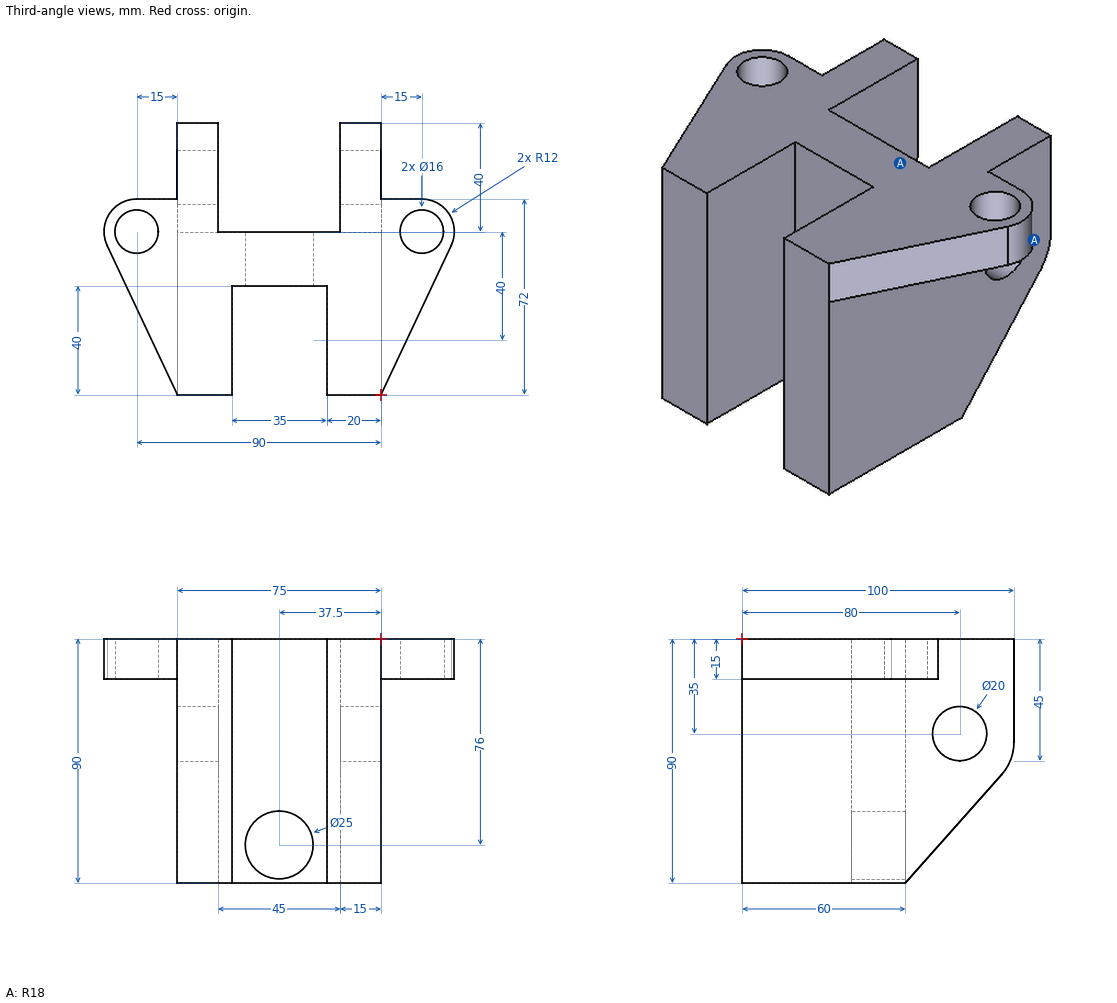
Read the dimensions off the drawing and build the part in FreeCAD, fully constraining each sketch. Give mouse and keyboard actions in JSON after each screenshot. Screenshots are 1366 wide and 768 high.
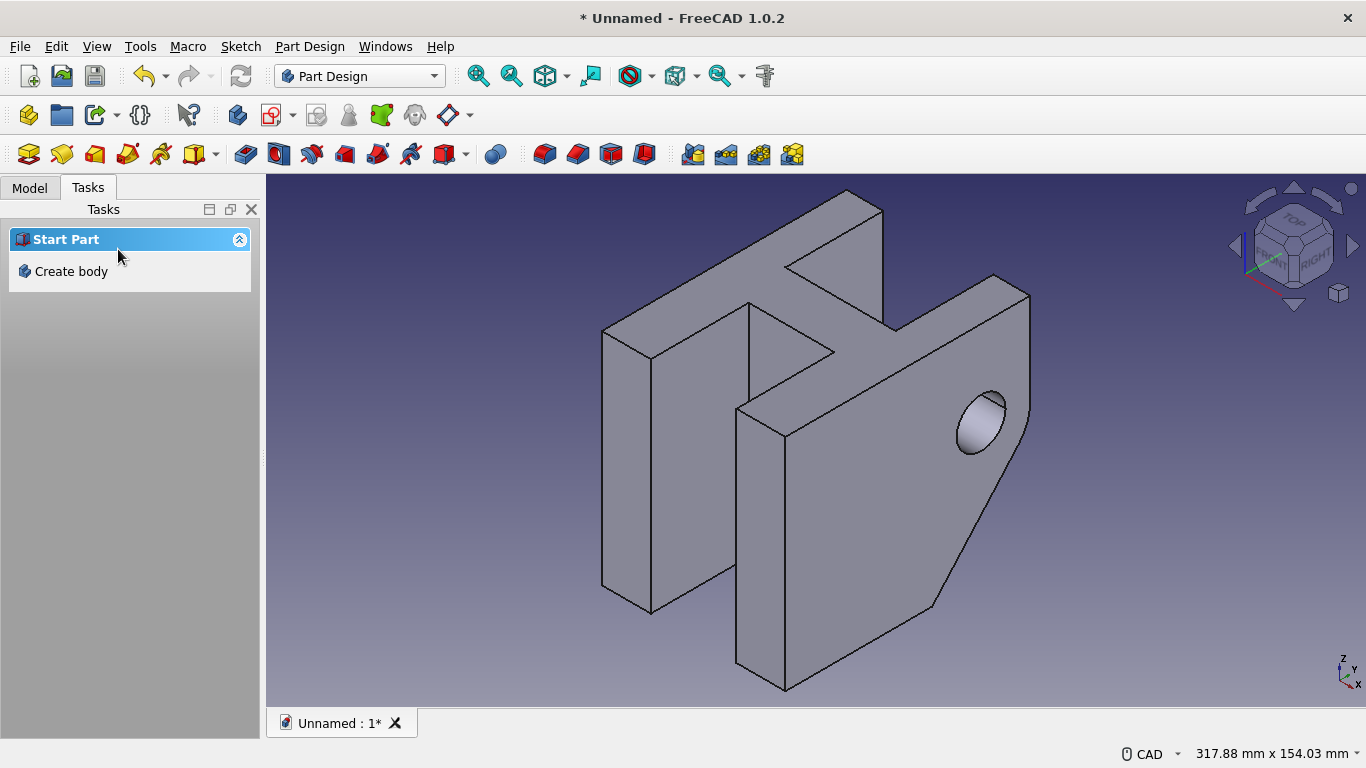
{"action": "key", "text": "4"}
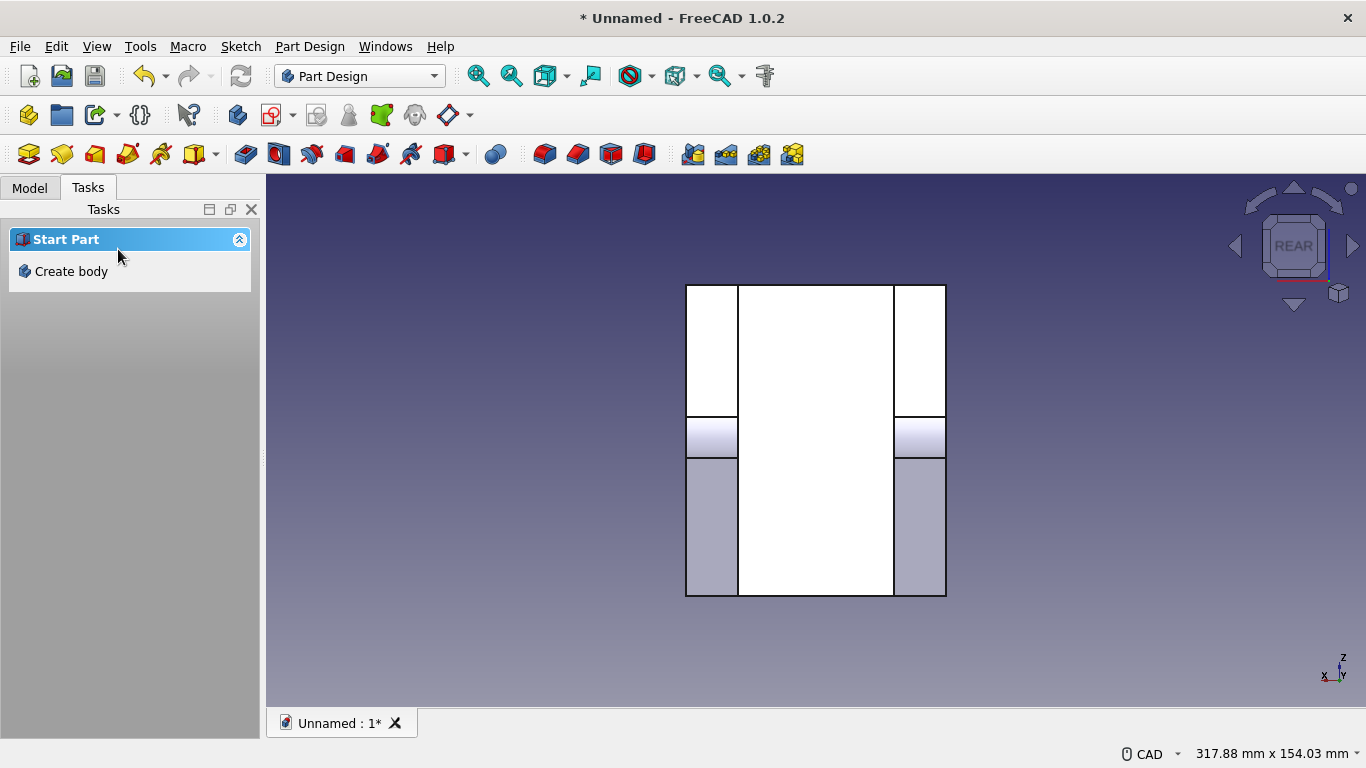
{"action": "left_click", "coordinate": [816, 484]}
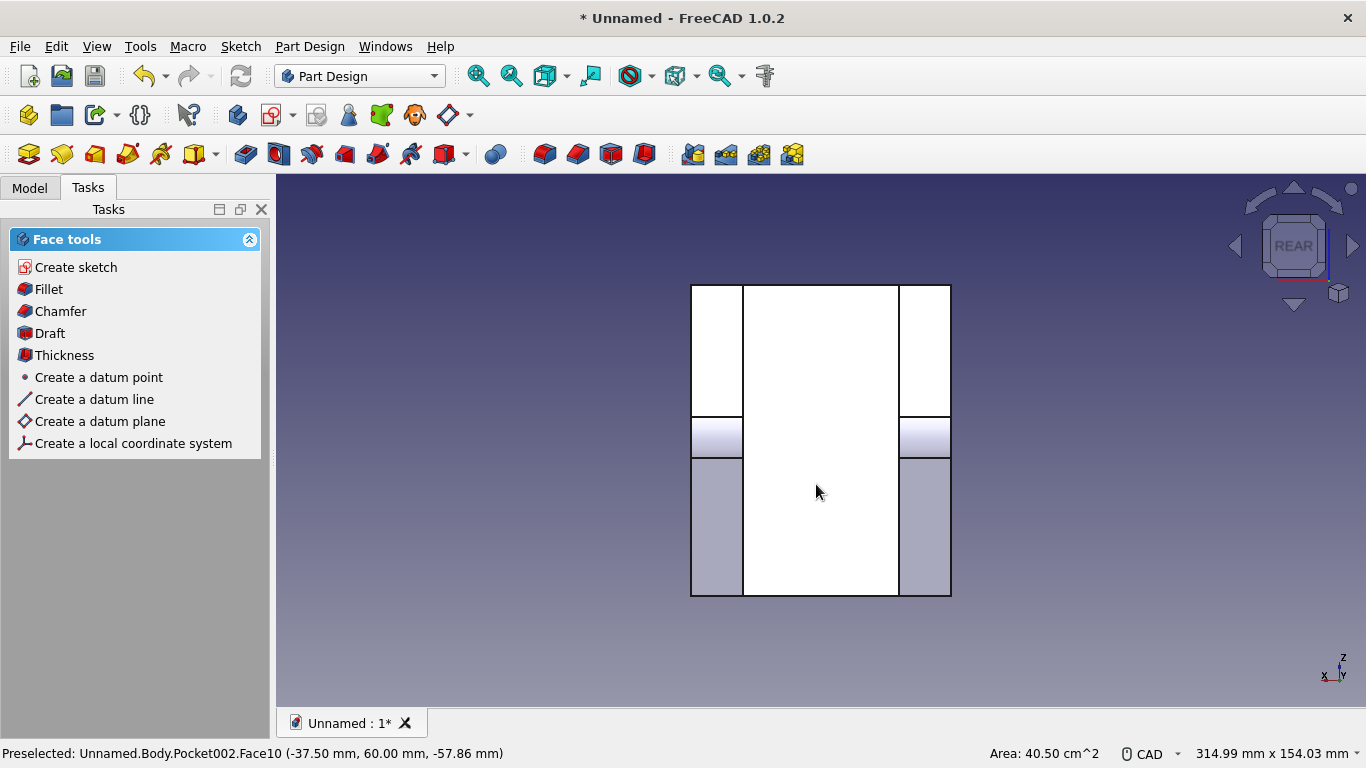
{"action": "left_click", "coordinate": [270, 116]}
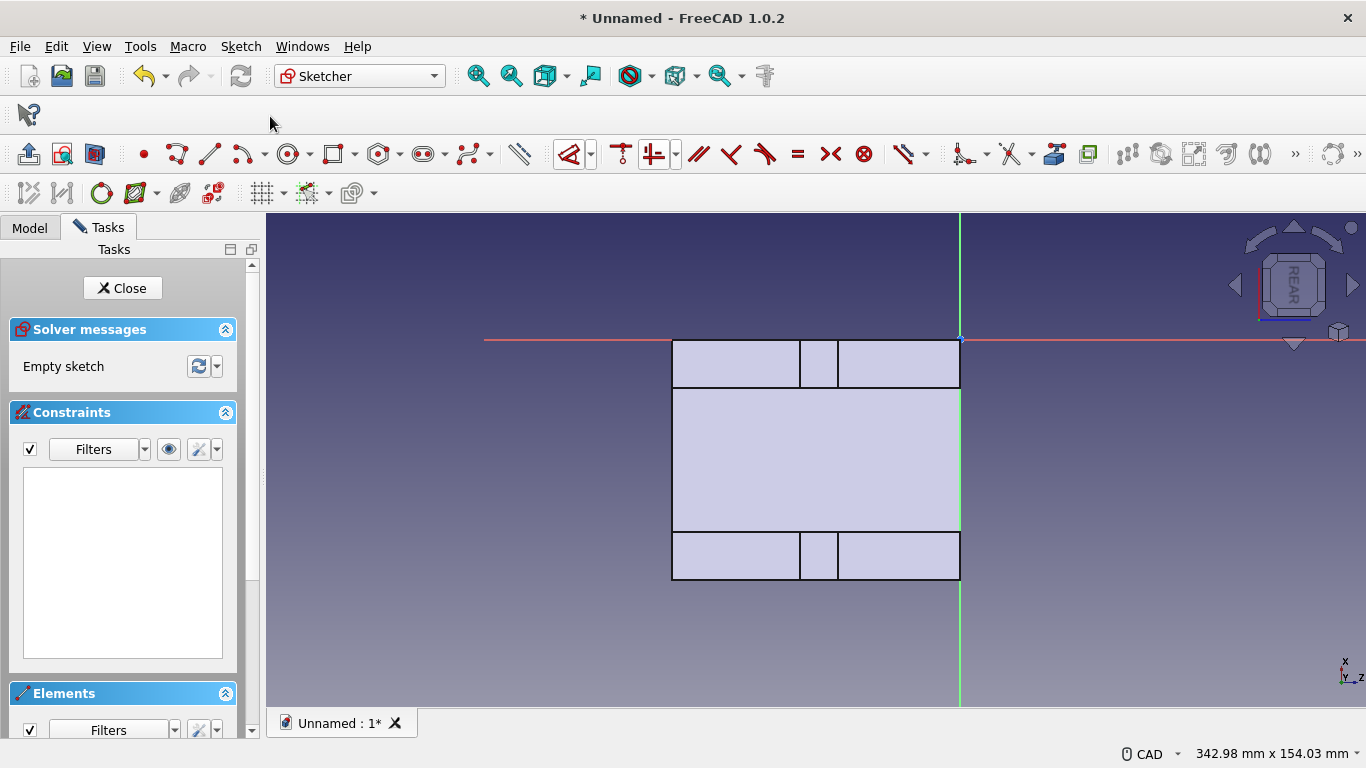
{"action": "scroll", "coordinate": [706, 460], "scroll_direction": "up", "scroll_amount": 7}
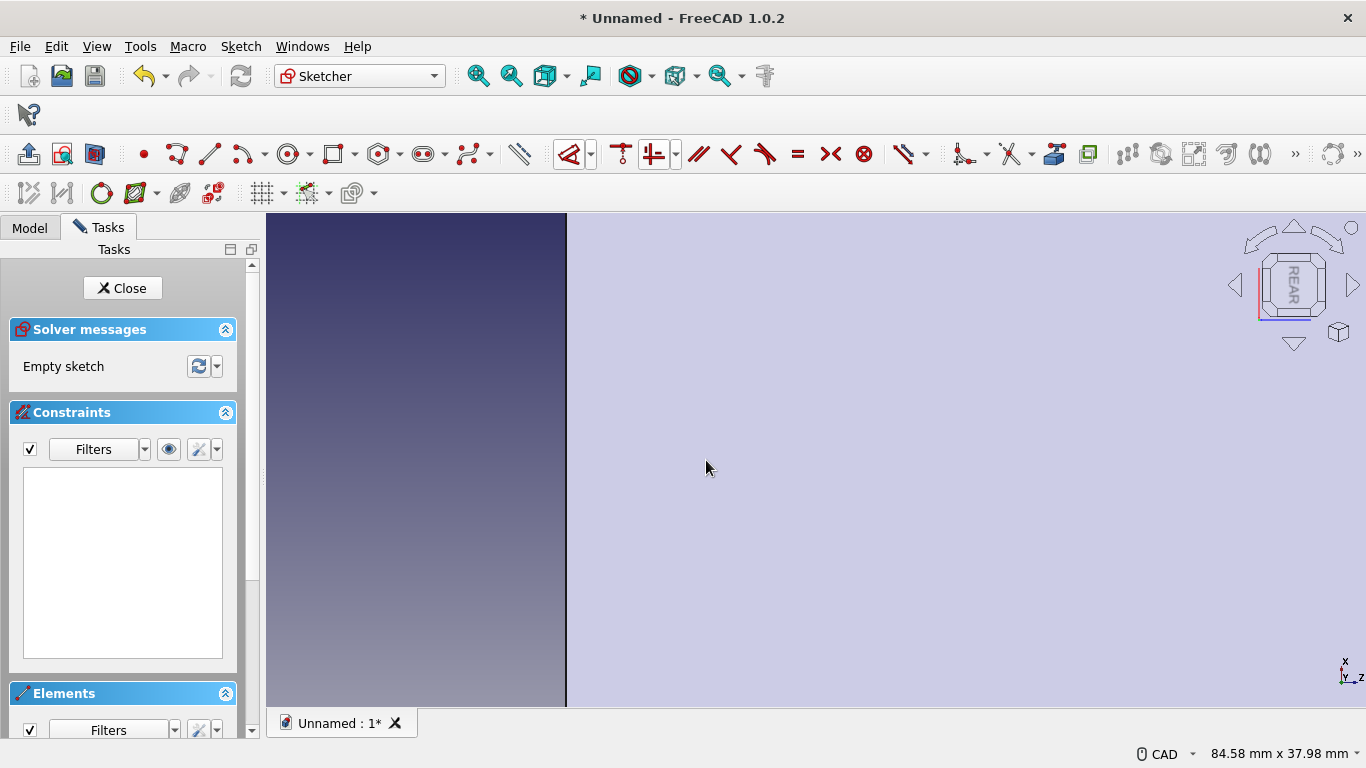
{"action": "left_click", "coordinate": [288, 154]}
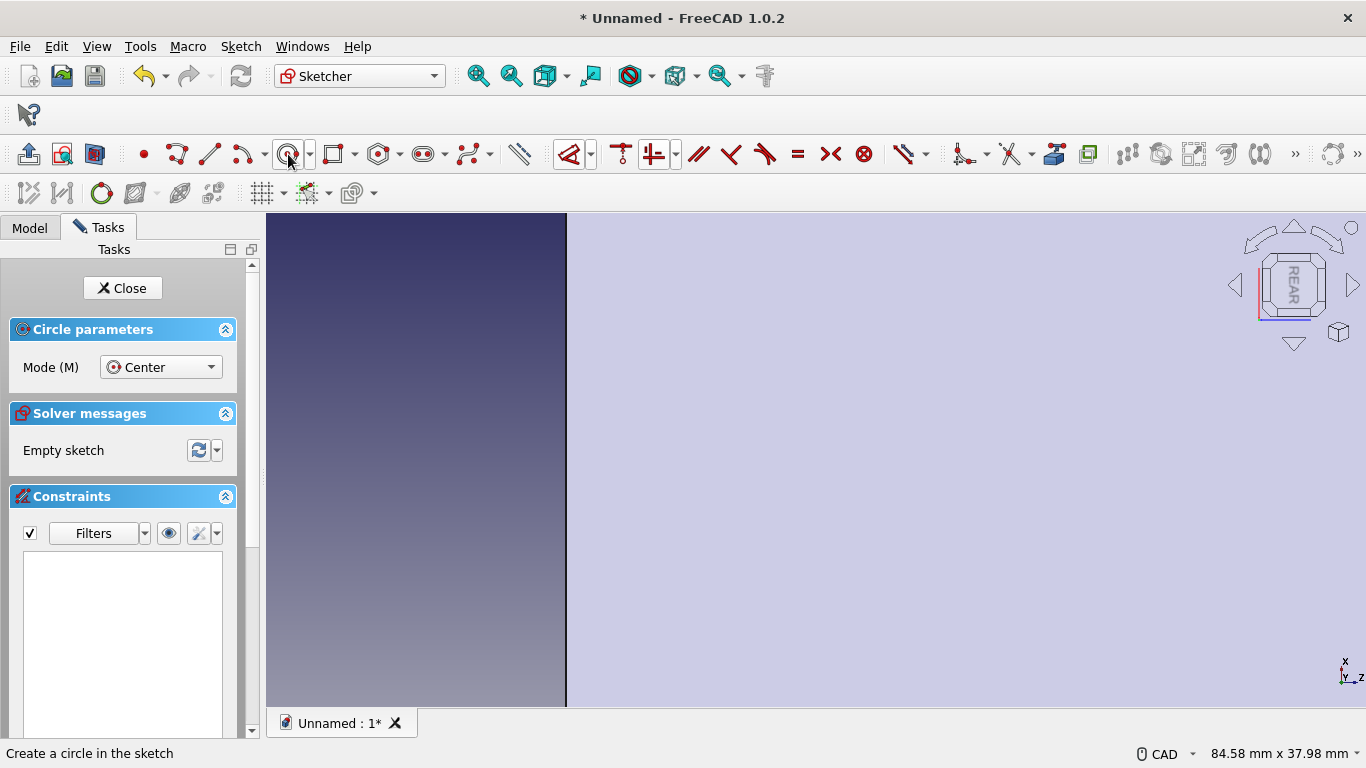
{"action": "left_click", "coordinate": [748, 458]}
{"action": "left_click", "coordinate": [863, 344]}
{"action": "key", "text": "Escape"}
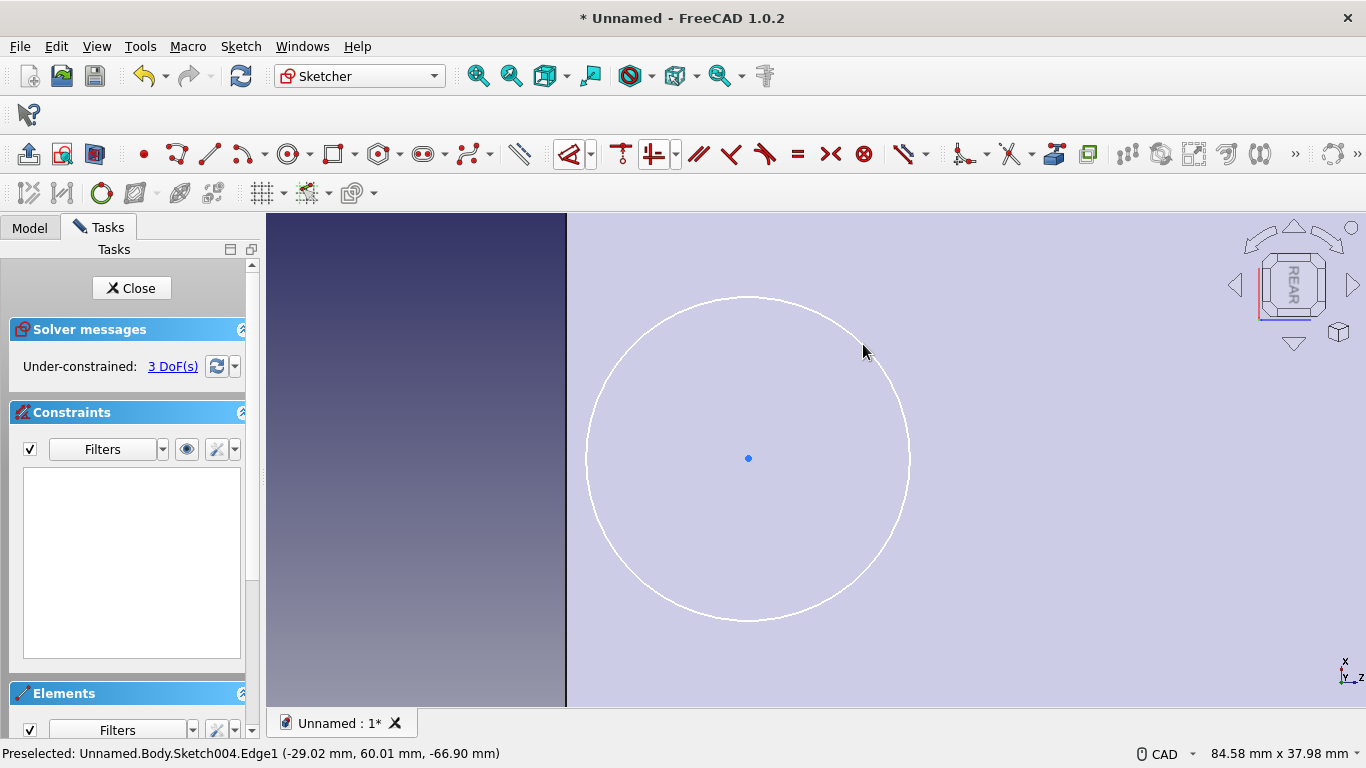
{"action": "left_click", "coordinate": [862, 344]}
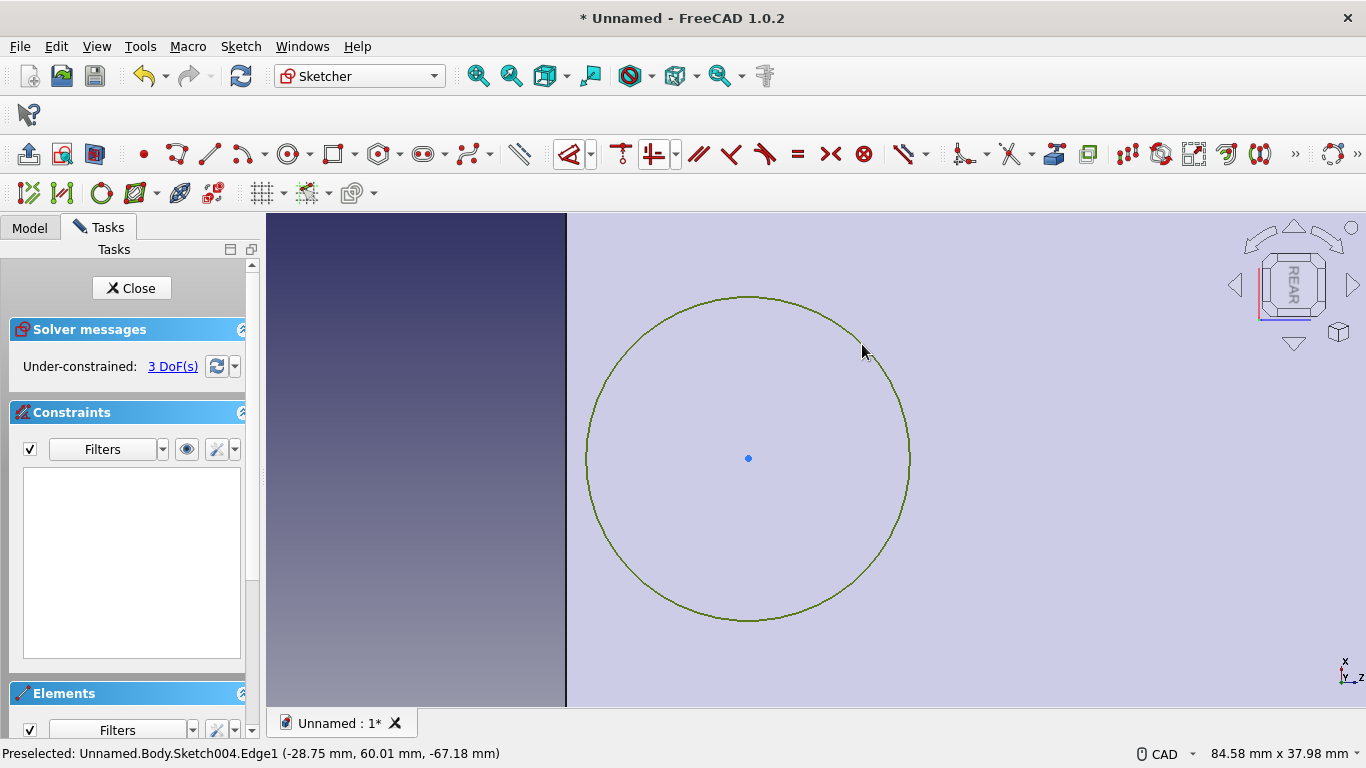
{"action": "left_click", "coordinate": [590, 154]}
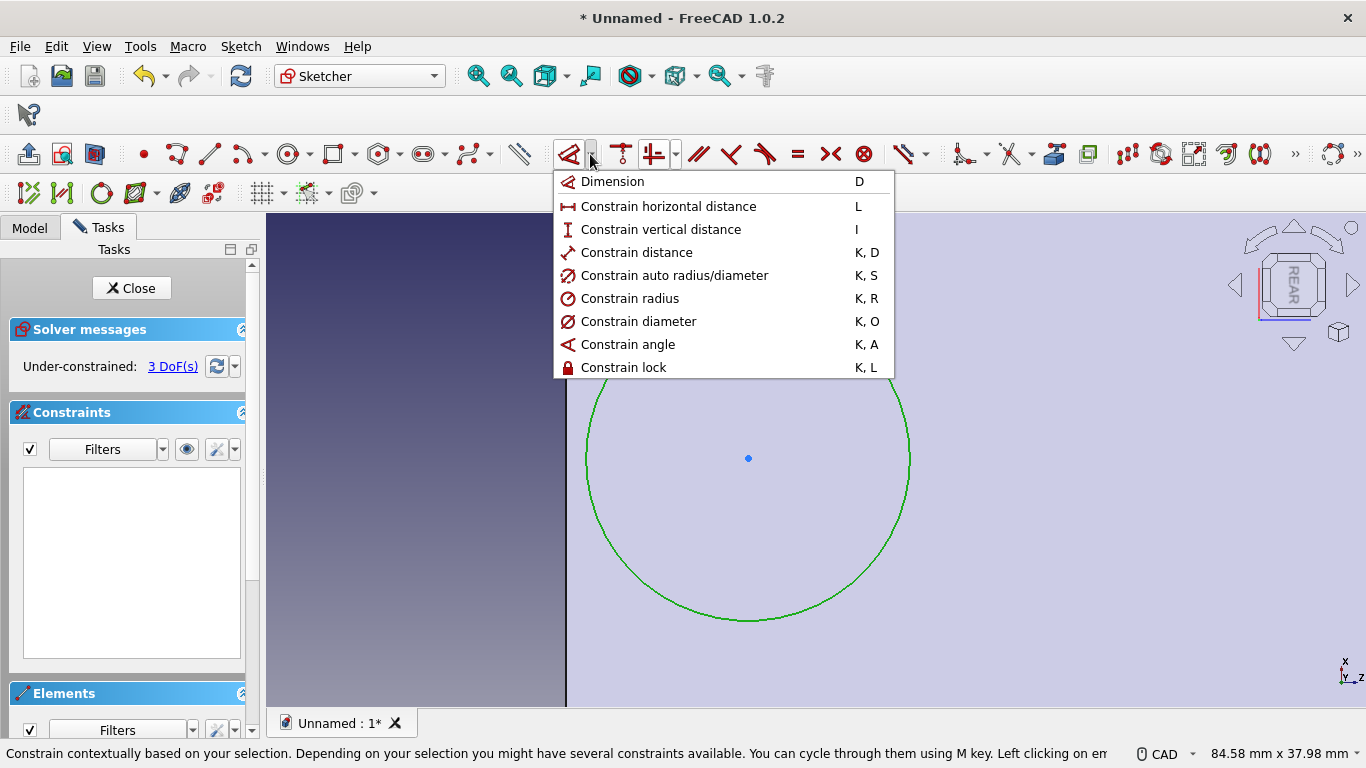
{"action": "left_click", "coordinate": [724, 322]}